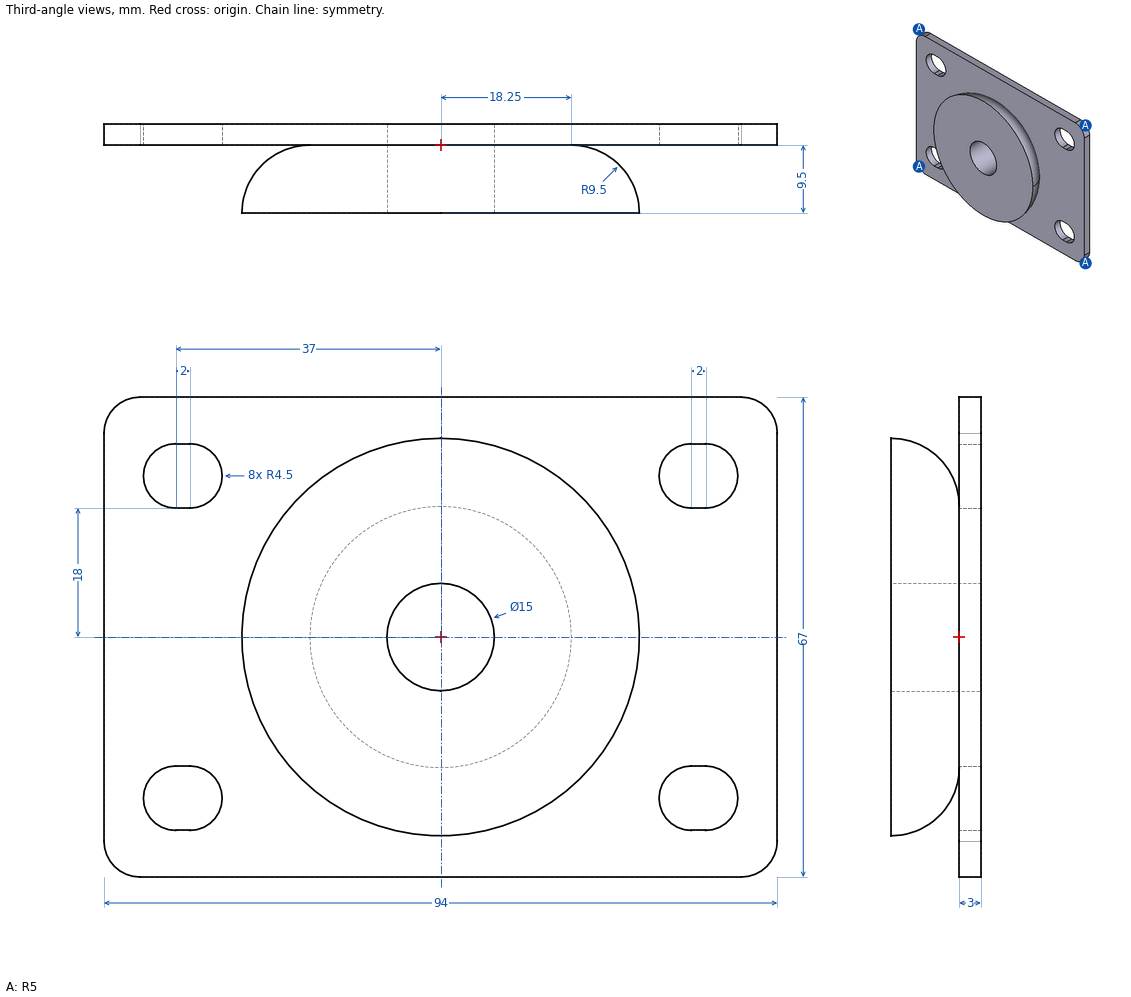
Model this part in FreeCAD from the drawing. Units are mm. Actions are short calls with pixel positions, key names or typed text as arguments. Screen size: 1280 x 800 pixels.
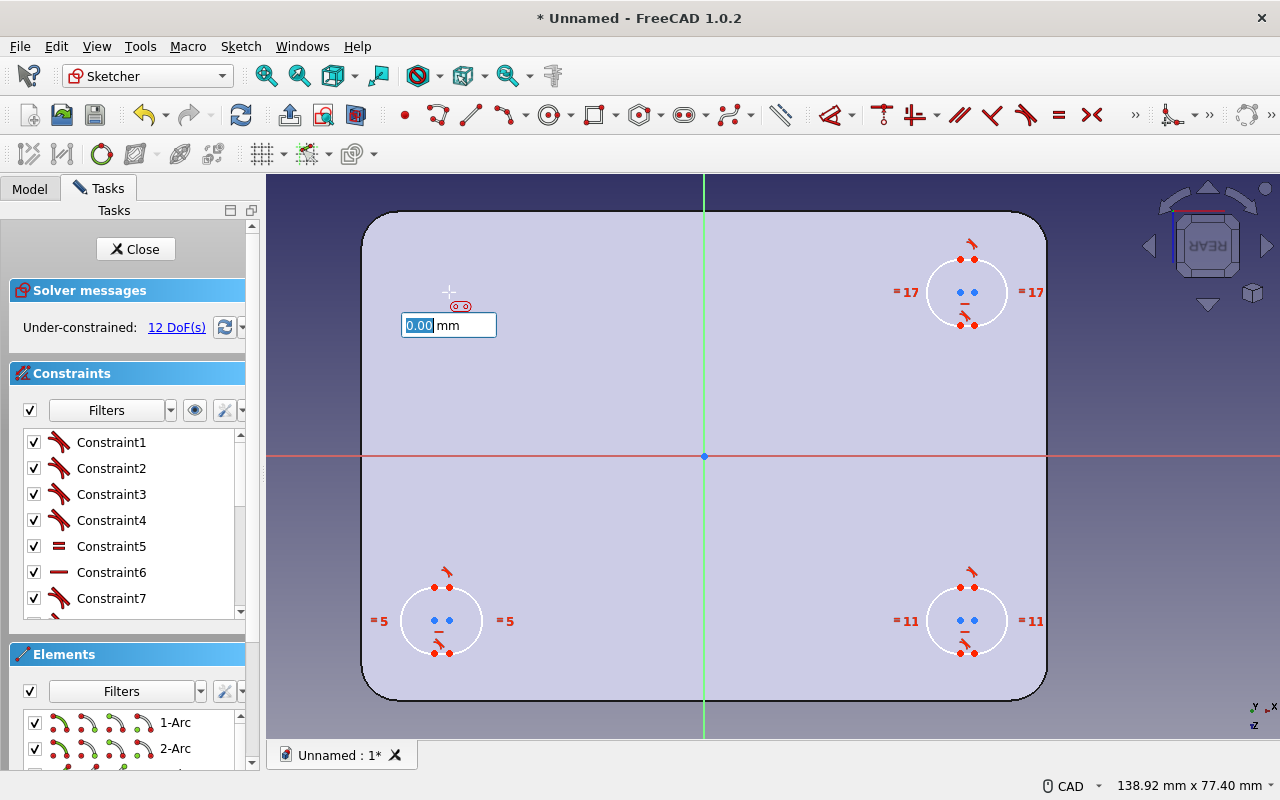
click(442, 325)
key(Escape)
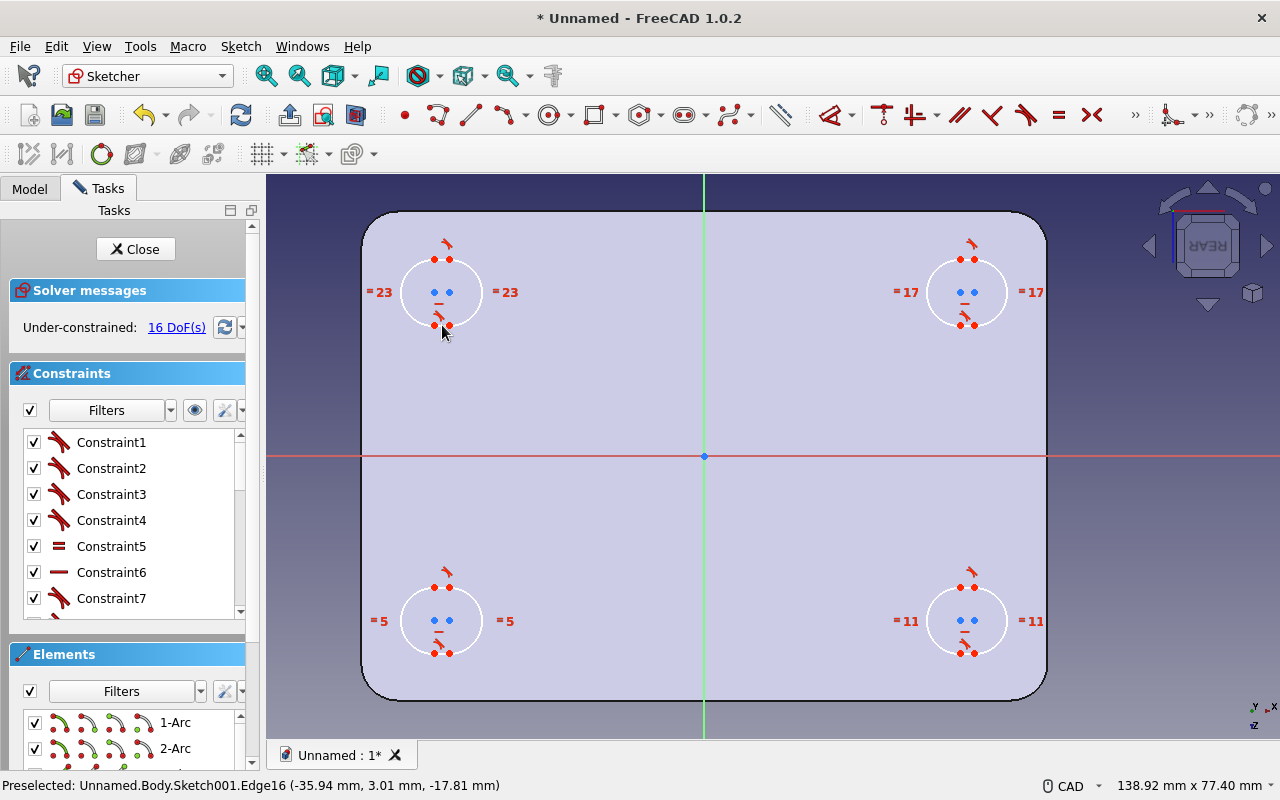
click(407, 602)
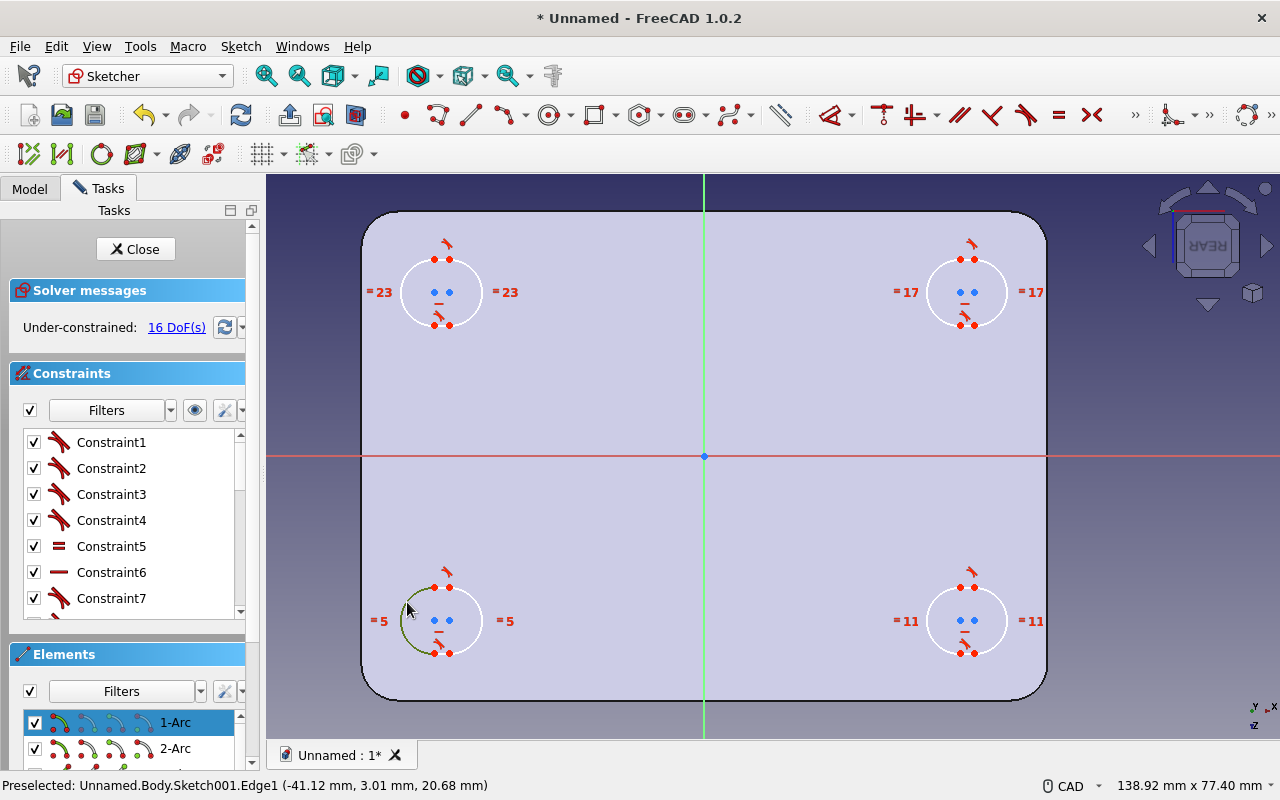
click(933, 602)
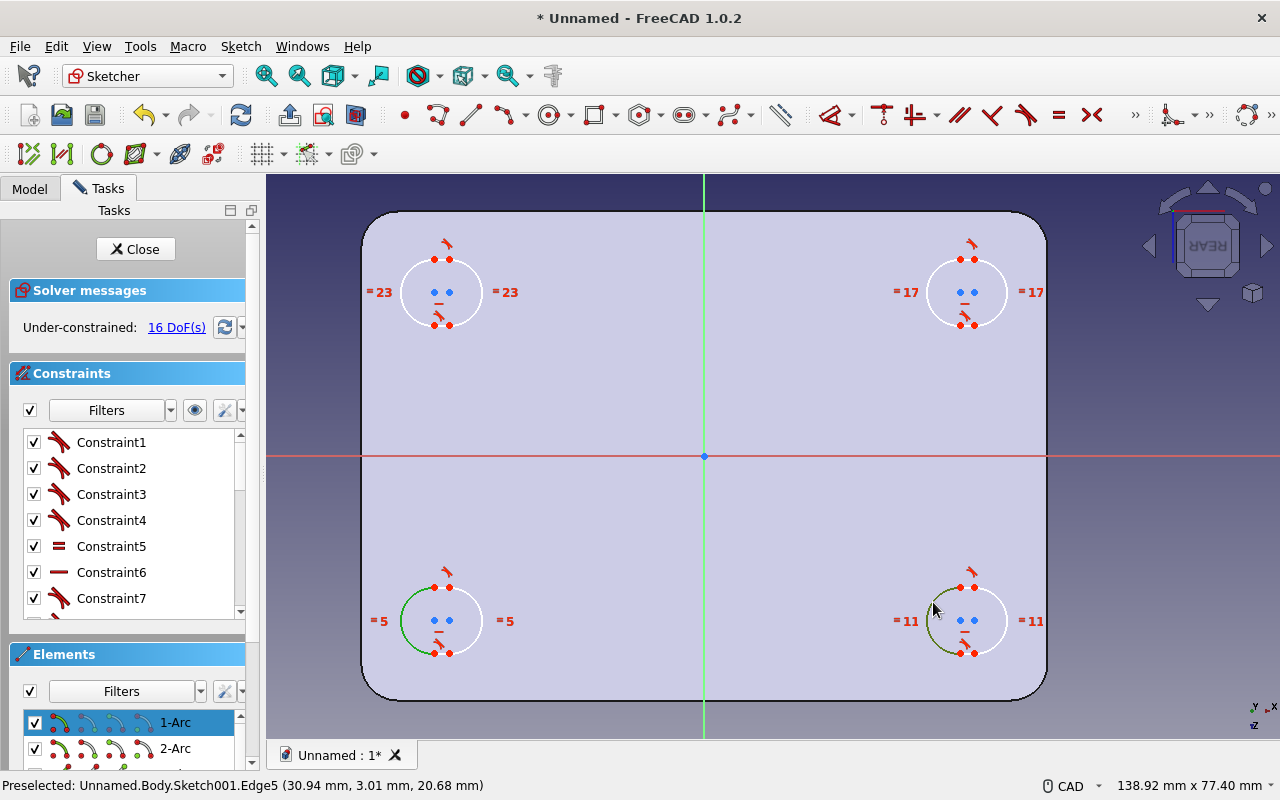
click(933, 274)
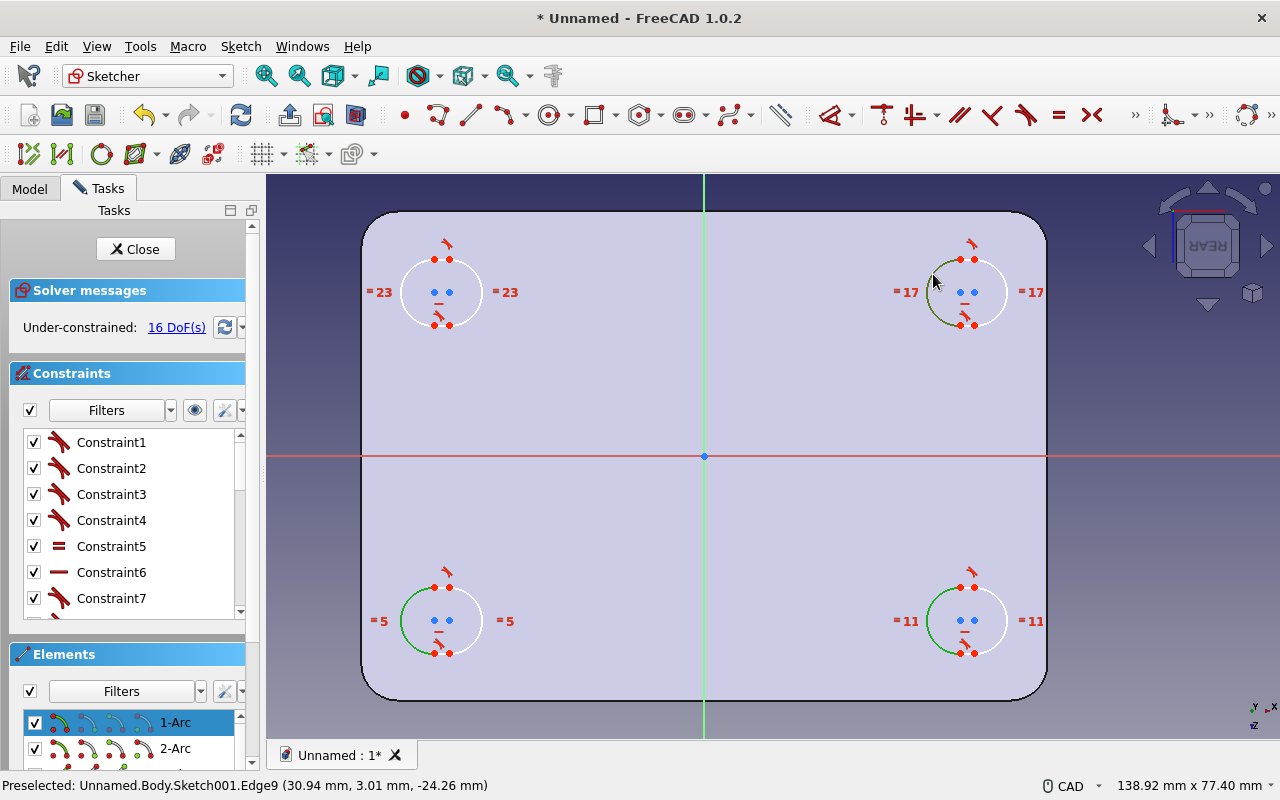
click(407, 274)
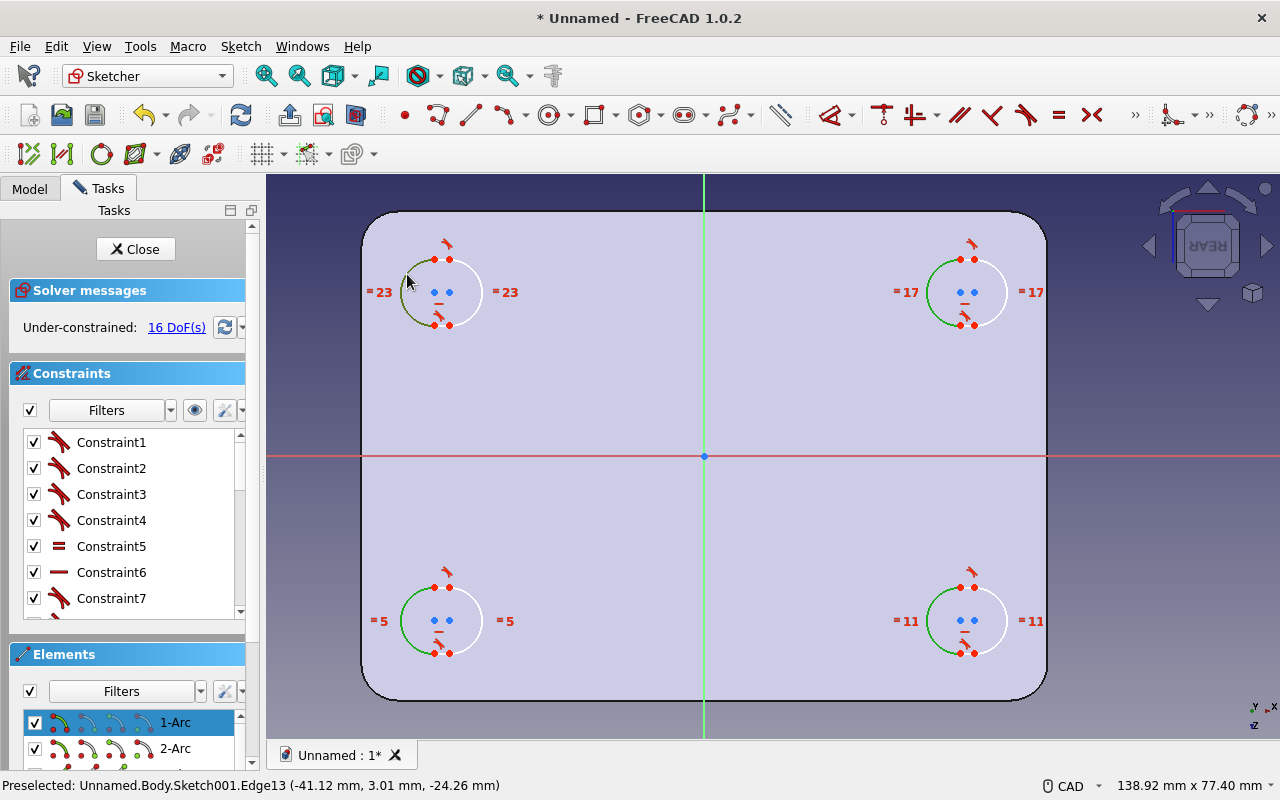
click(1059, 116)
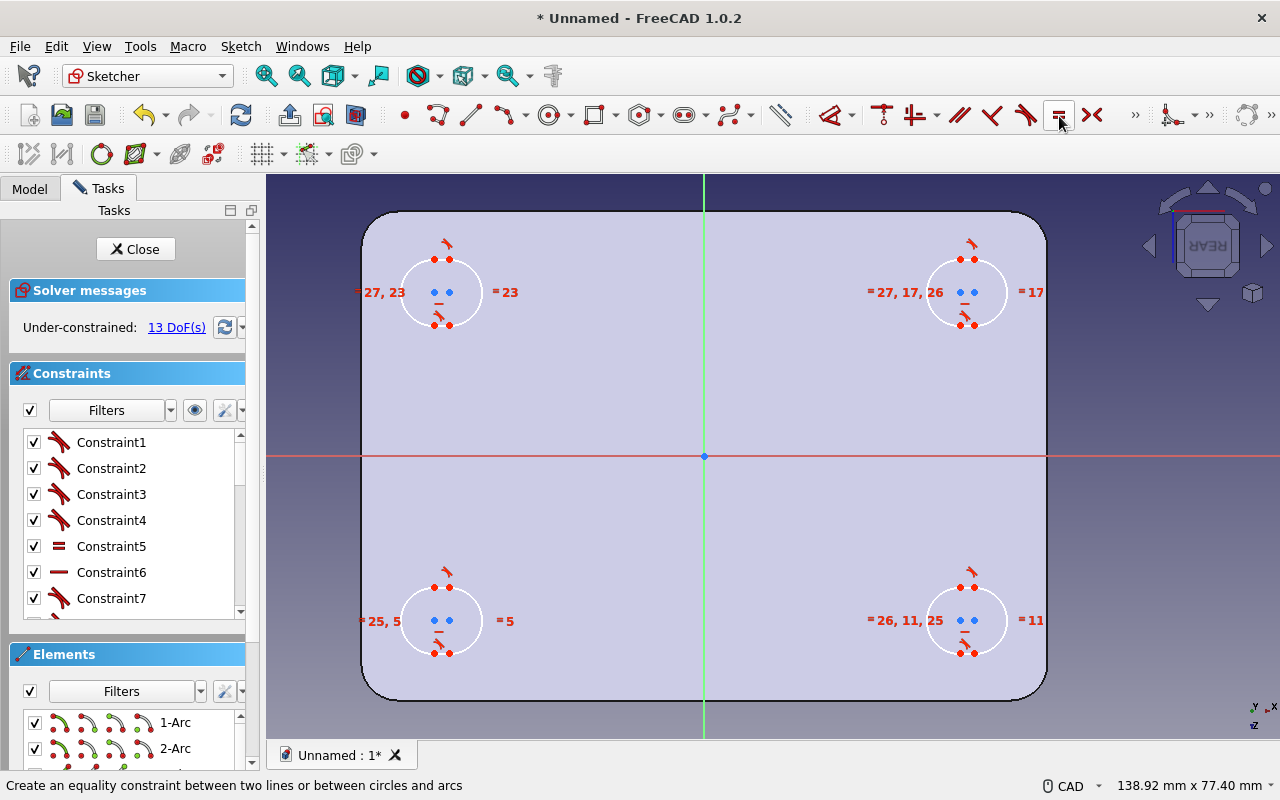
click(449, 621)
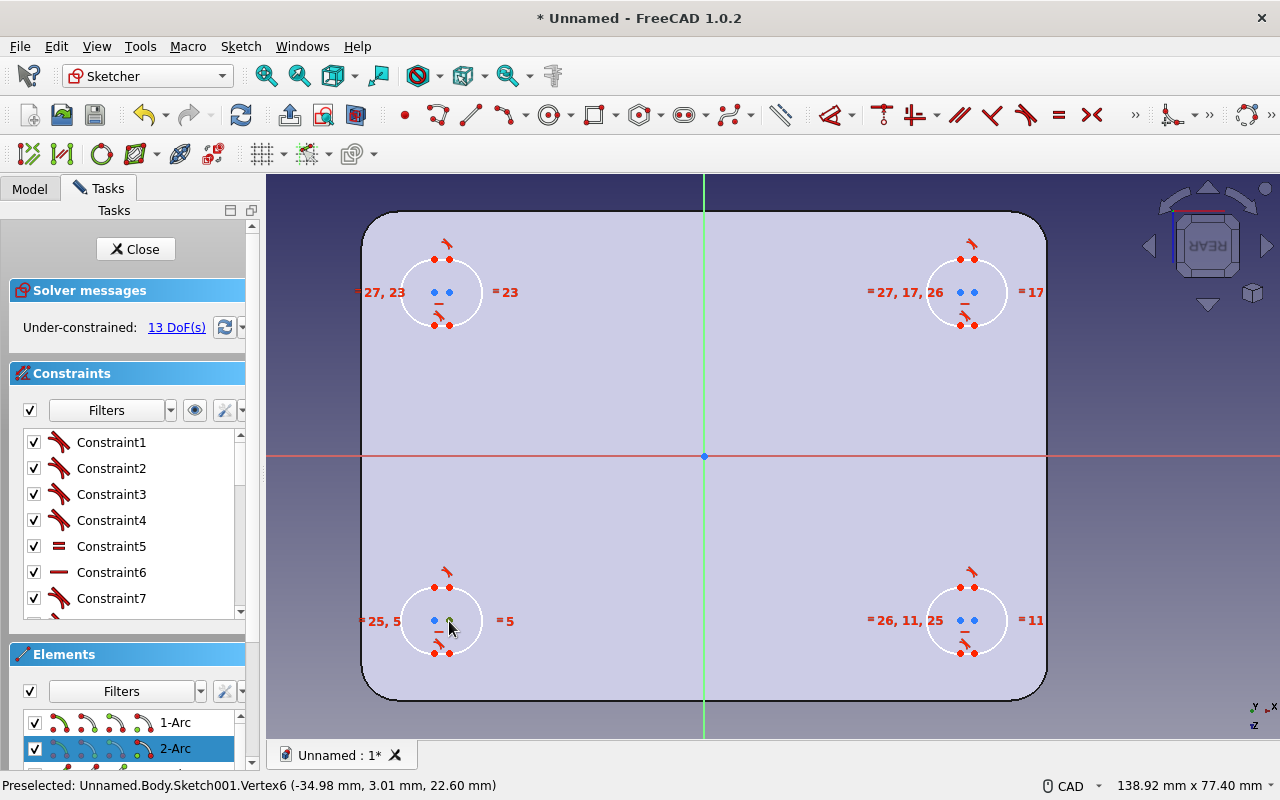
click(960, 621)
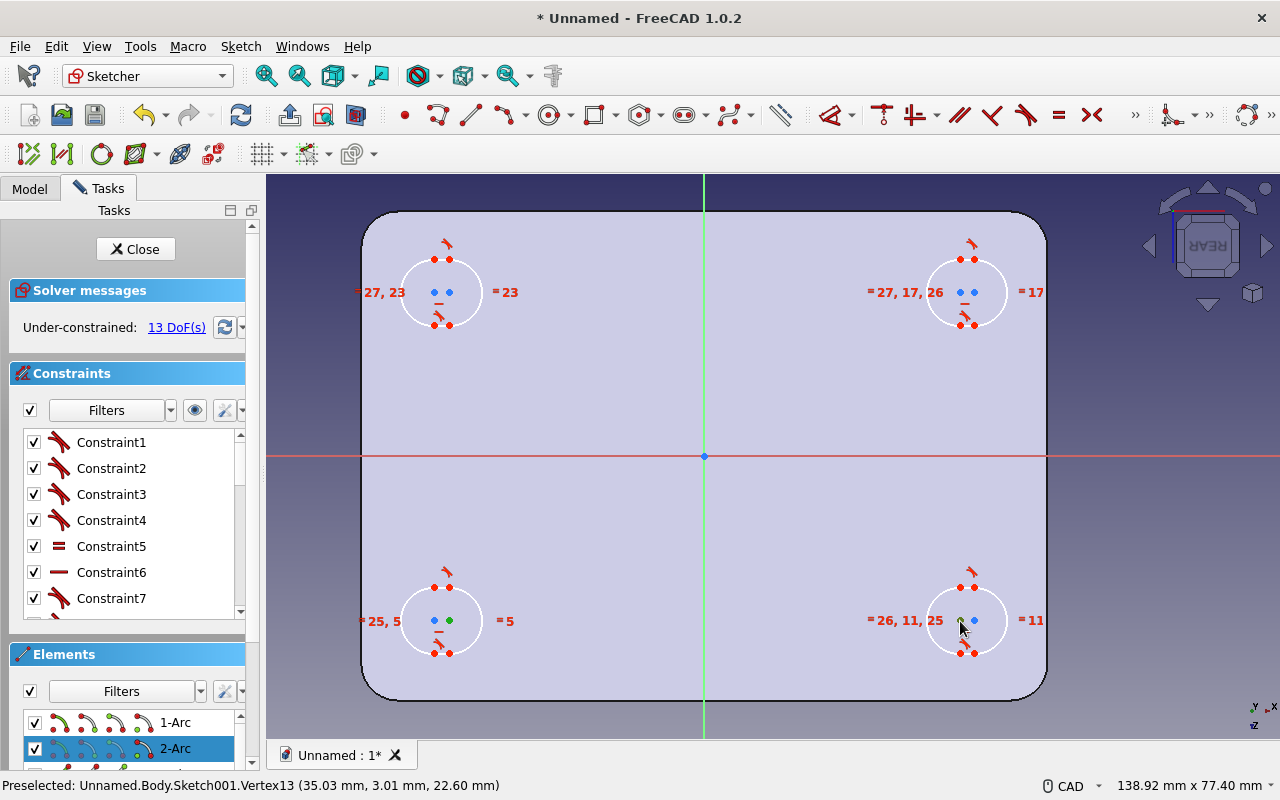
click(704, 675)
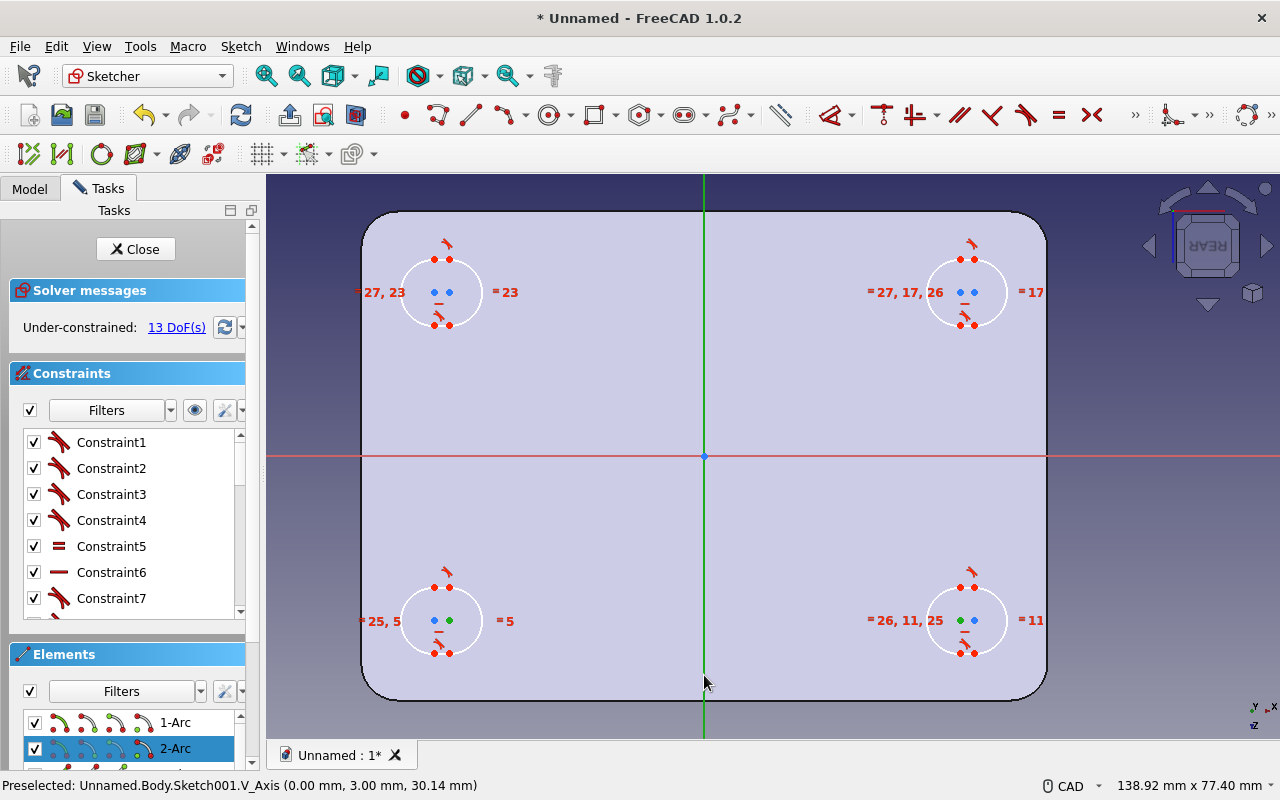
key(s)